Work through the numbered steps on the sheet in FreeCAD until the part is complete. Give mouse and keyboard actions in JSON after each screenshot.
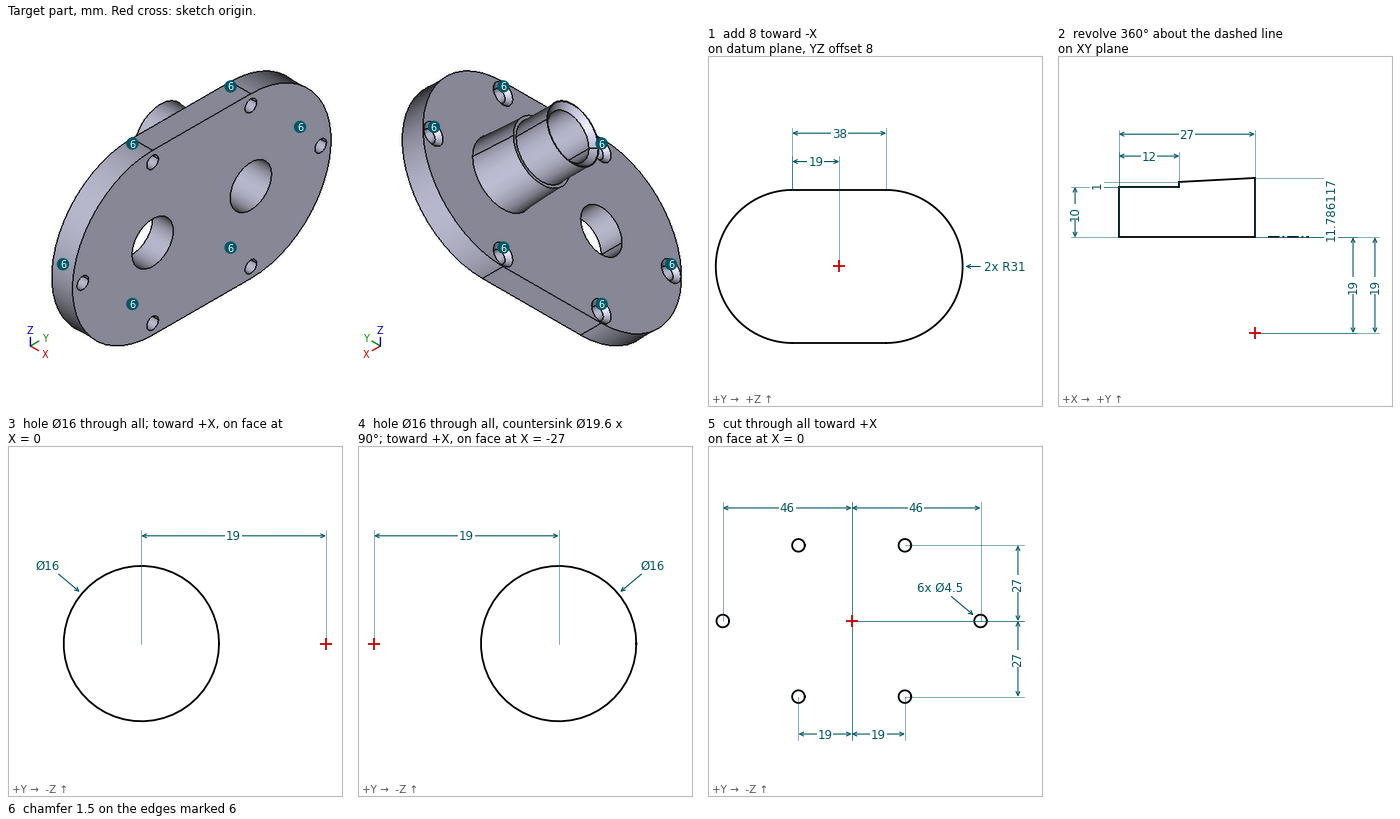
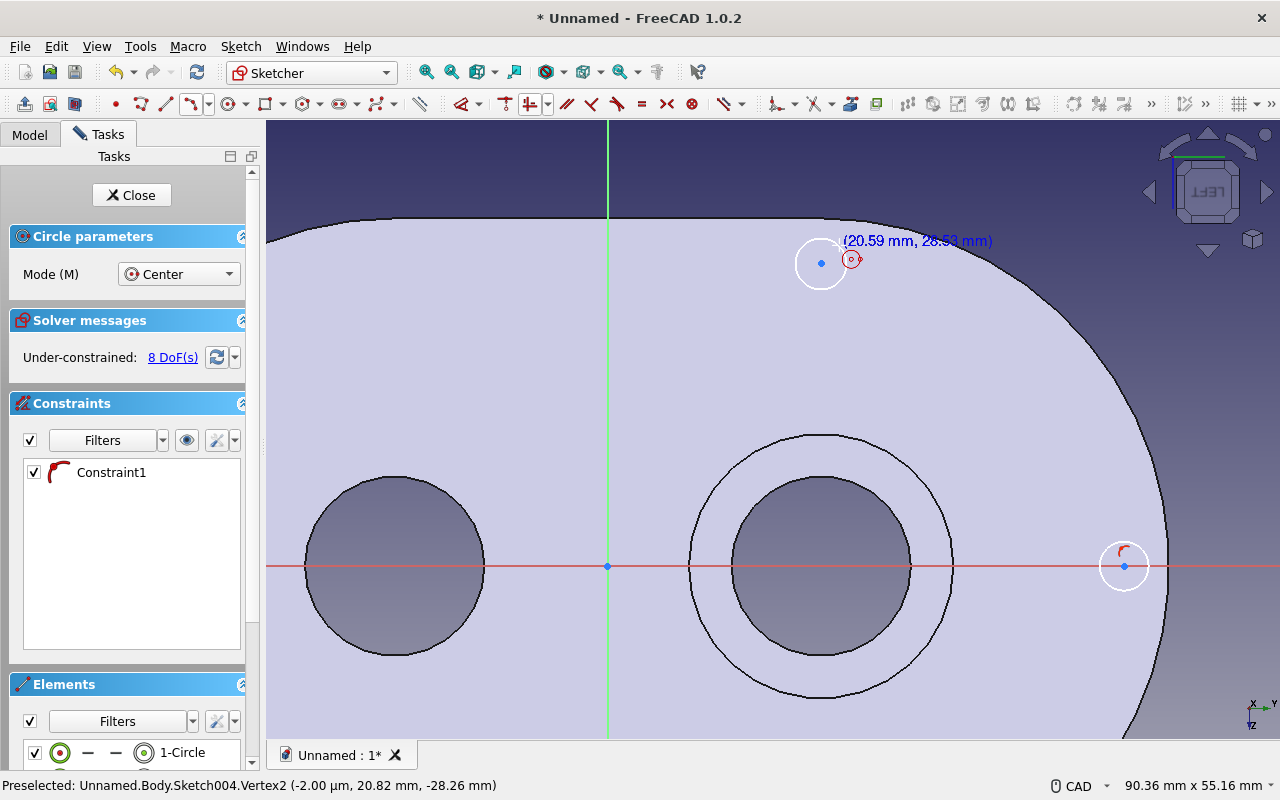
{"action": "scroll", "coordinate": [822, 263], "scroll_direction": "down", "scroll_amount": 3}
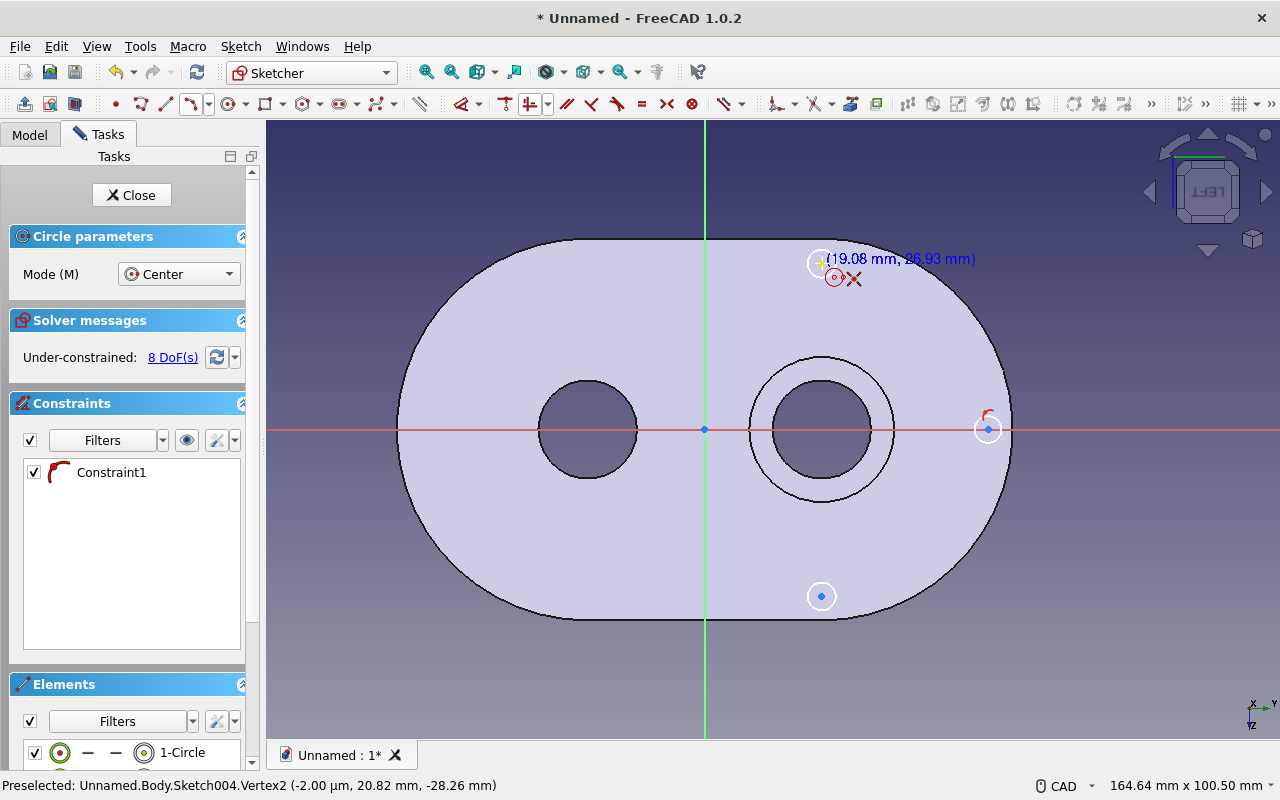
{"action": "scroll", "coordinate": [588, 596], "scroll_direction": "up", "scroll_amount": 3}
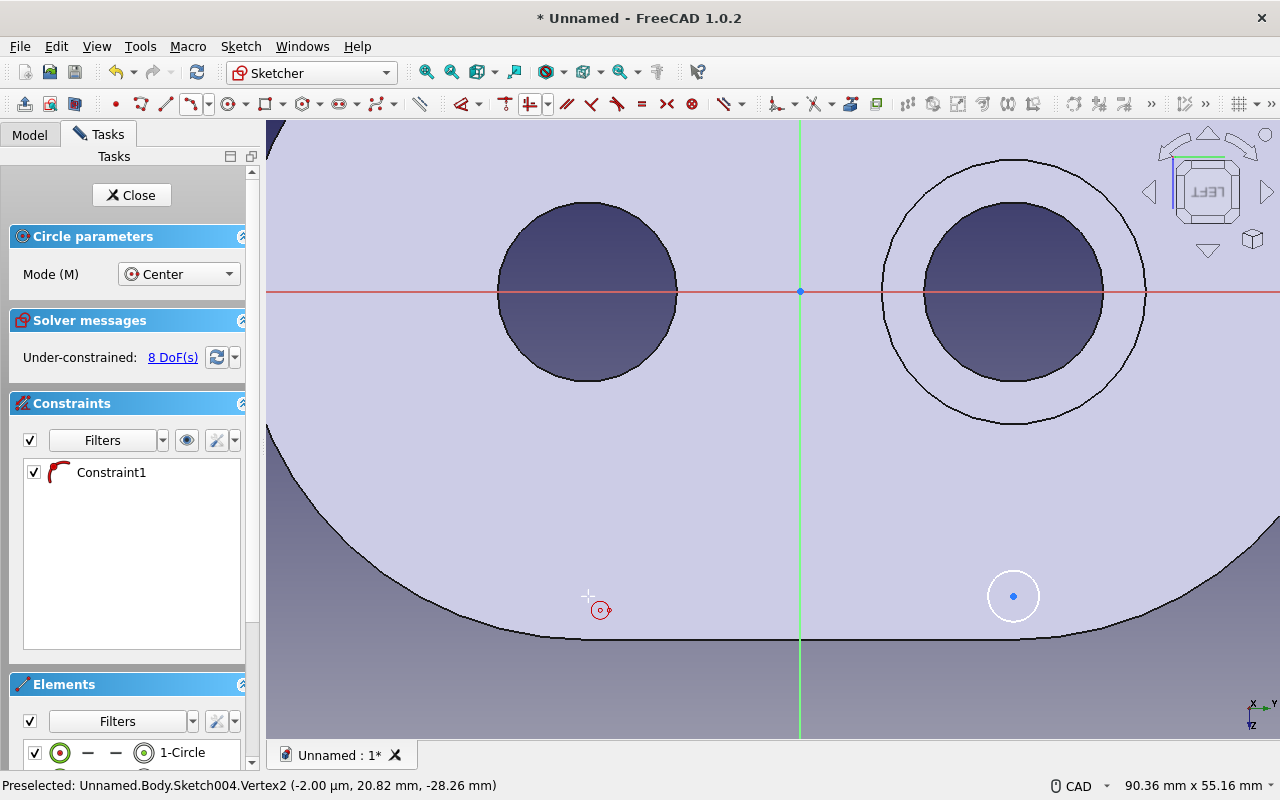
{"action": "left_click", "coordinate": [587, 595]}
{"action": "left_click", "coordinate": [605, 577]}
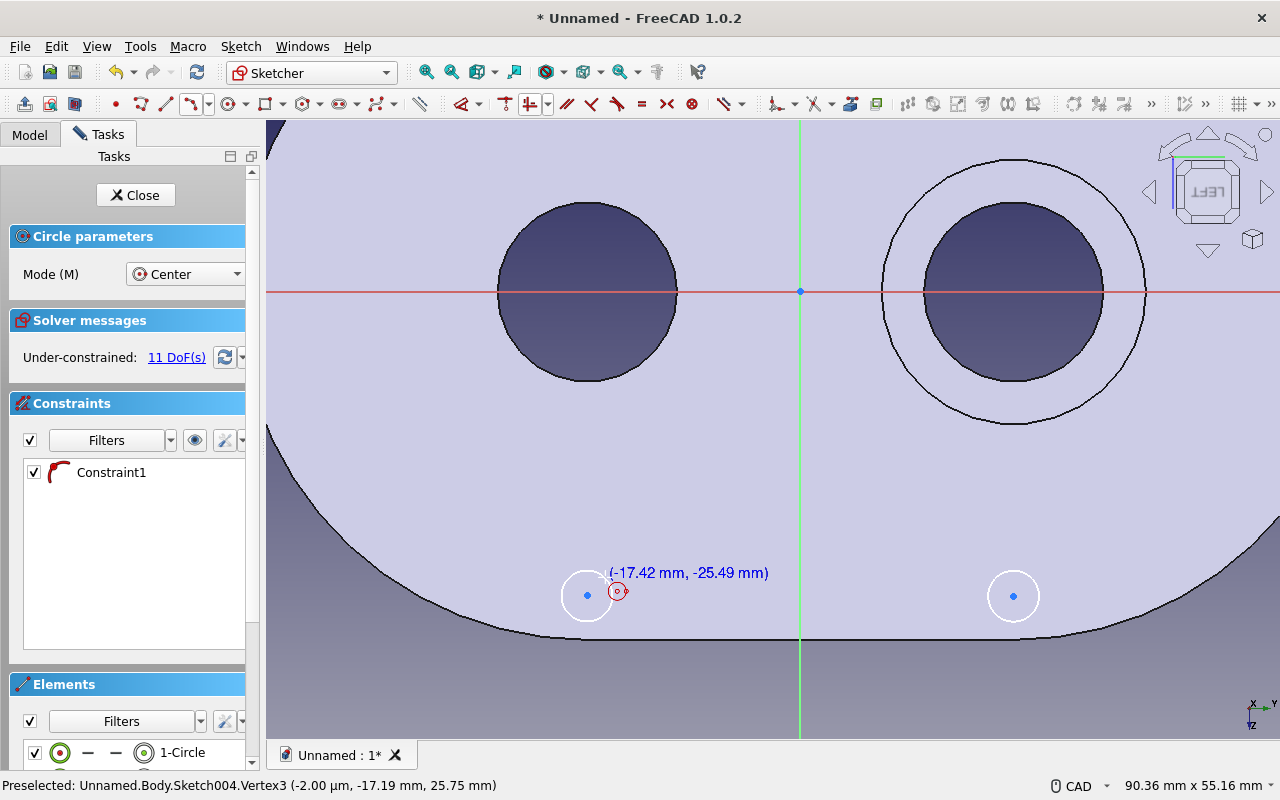
{"action": "scroll", "coordinate": [588, 597], "scroll_direction": "down", "scroll_amount": 3}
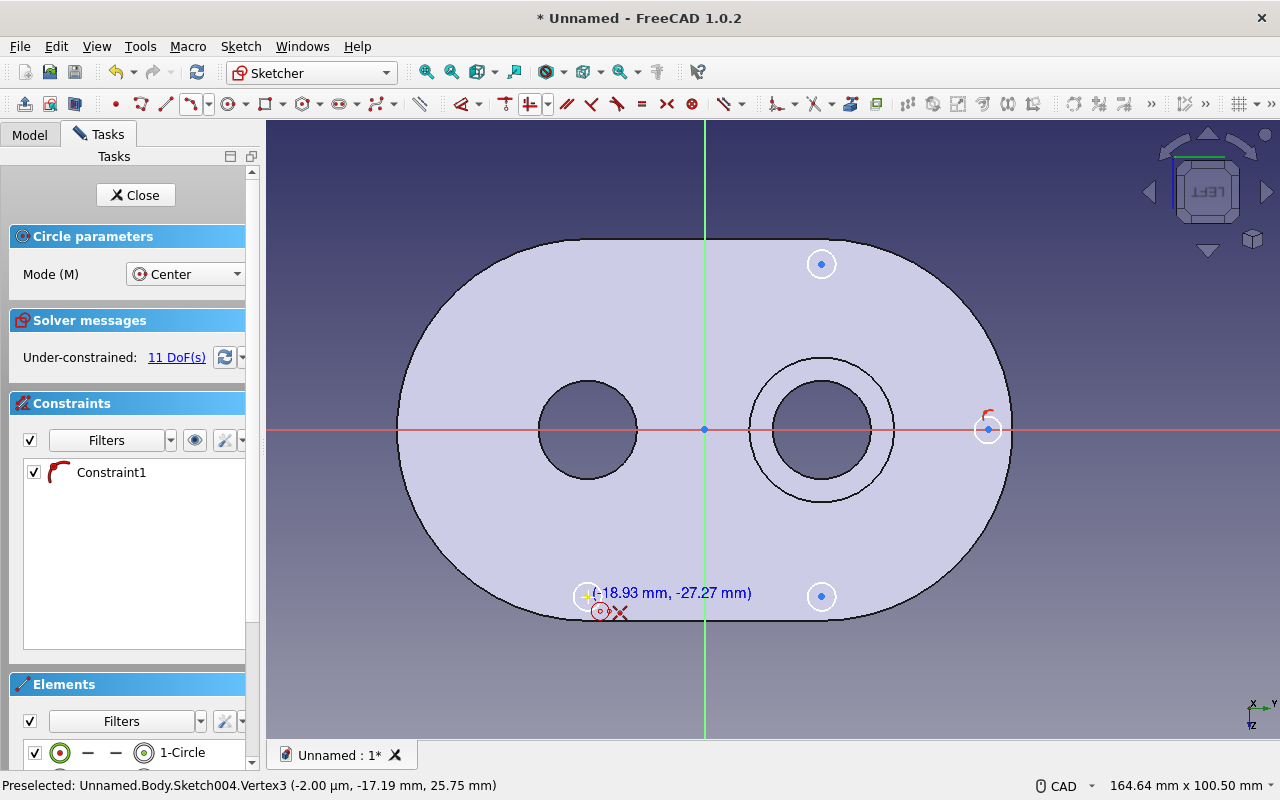
{"action": "scroll", "coordinate": [588, 264], "scroll_direction": "up", "scroll_amount": 3}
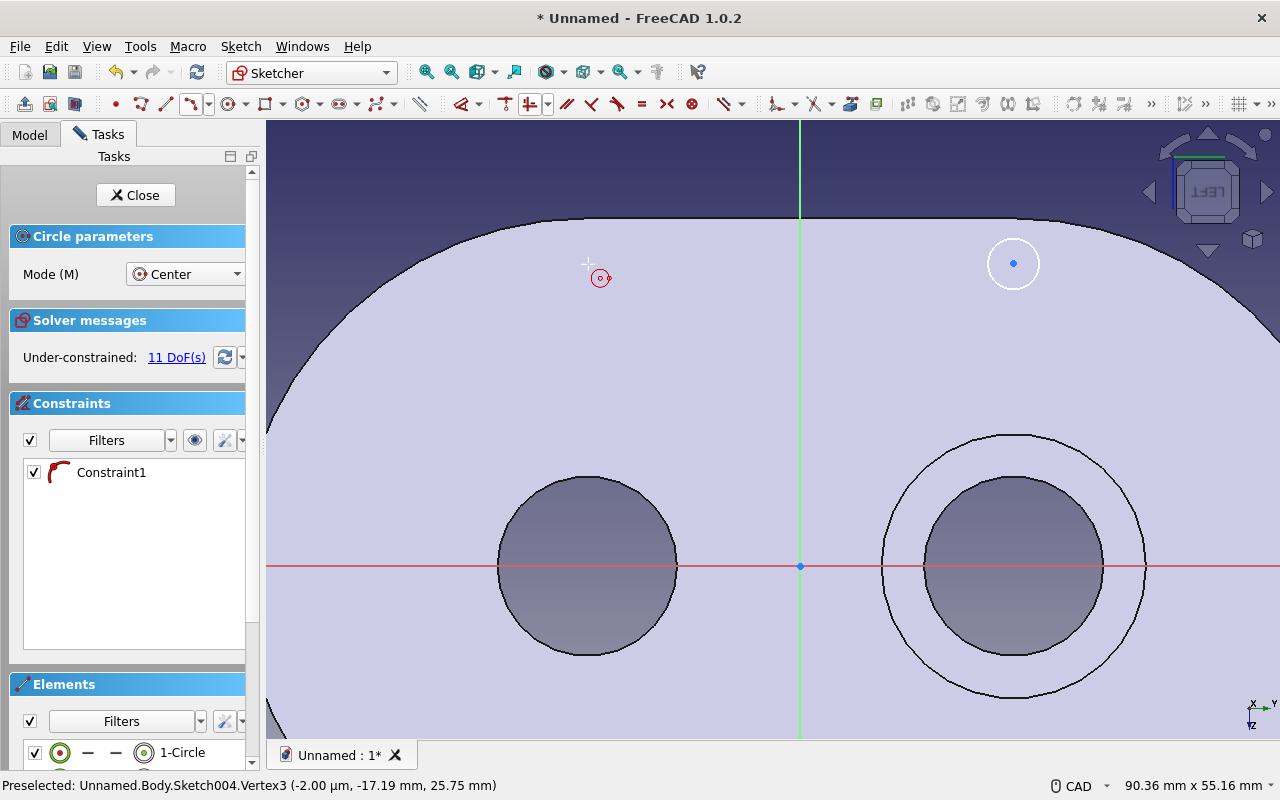
{"action": "left_click", "coordinate": [587, 263]}
{"action": "left_click", "coordinate": [605, 245]}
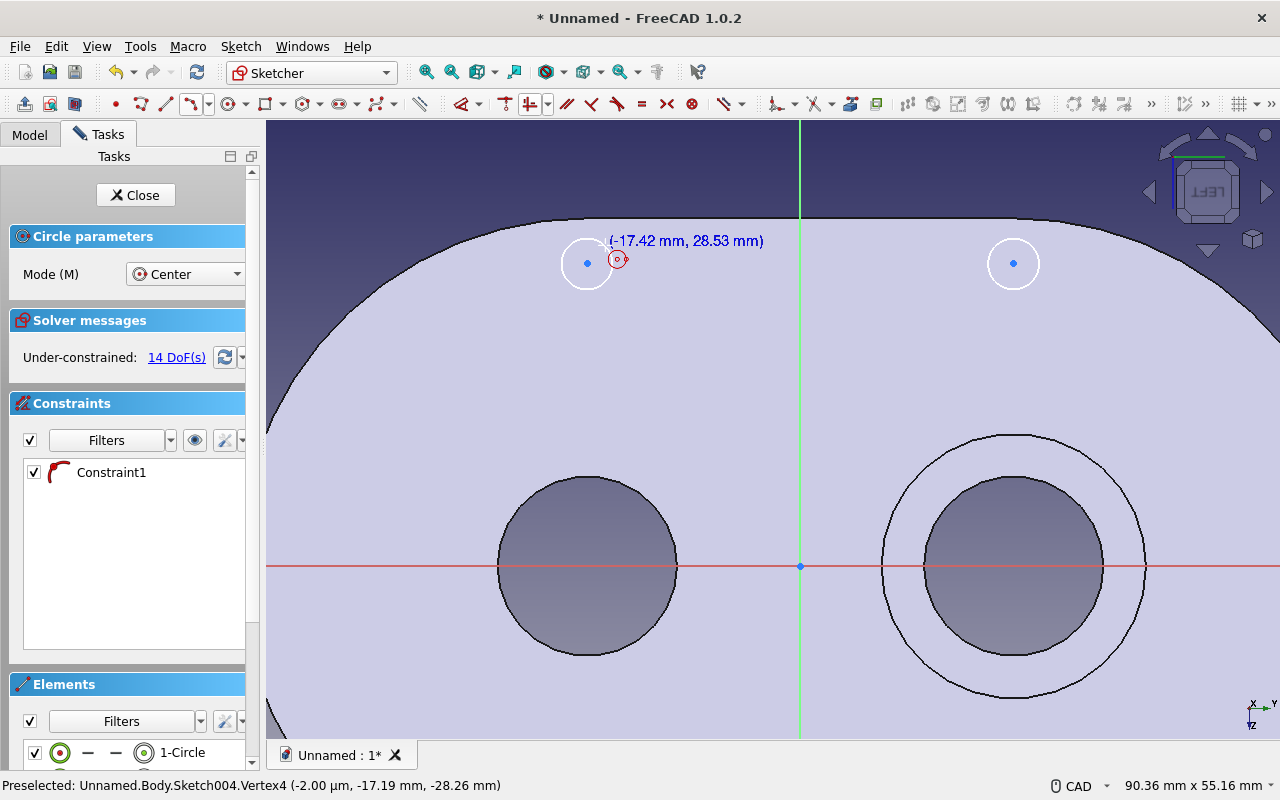
{"action": "scroll", "coordinate": [588, 263], "scroll_direction": "down", "scroll_amount": 3}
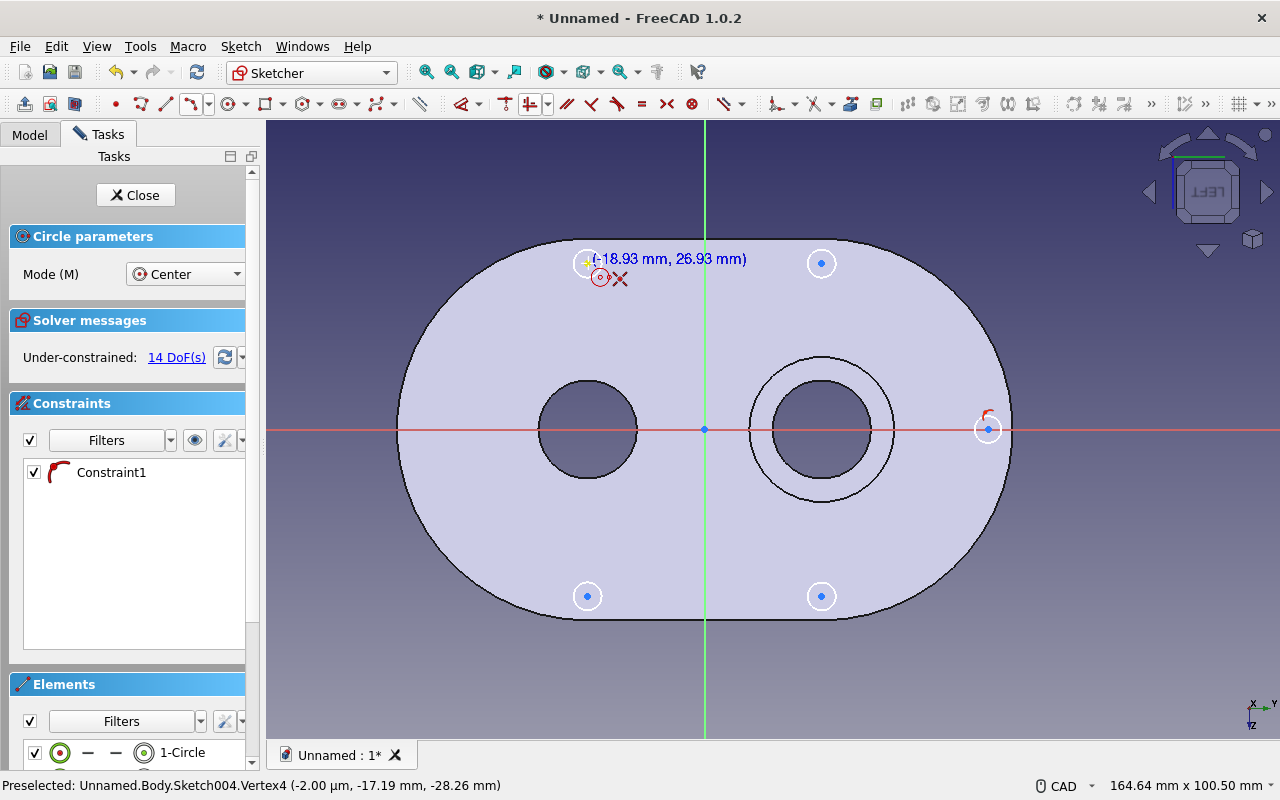
{"action": "scroll", "coordinate": [421, 429], "scroll_direction": "up", "scroll_amount": 3}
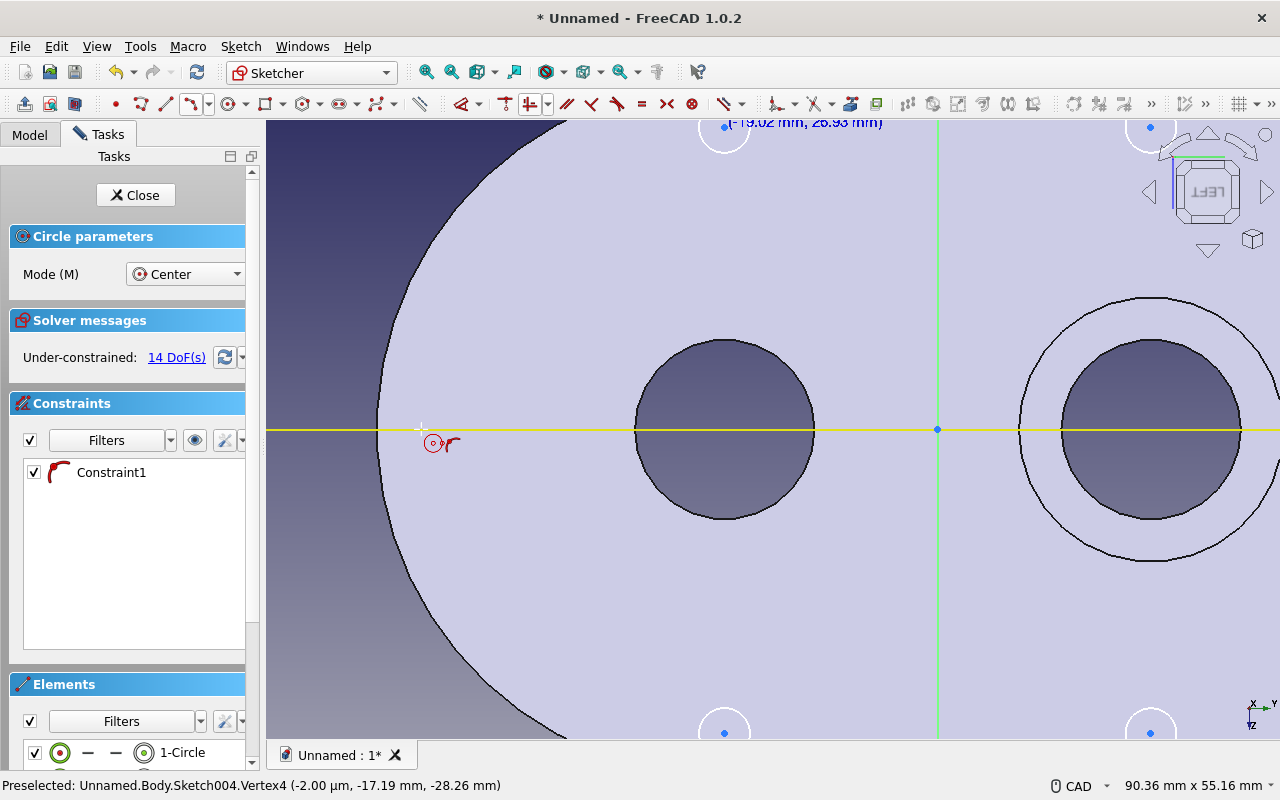
{"action": "left_click", "coordinate": [422, 429]}
{"action": "left_click", "coordinate": [440, 412]}
{"action": "key", "text": "Escape"}